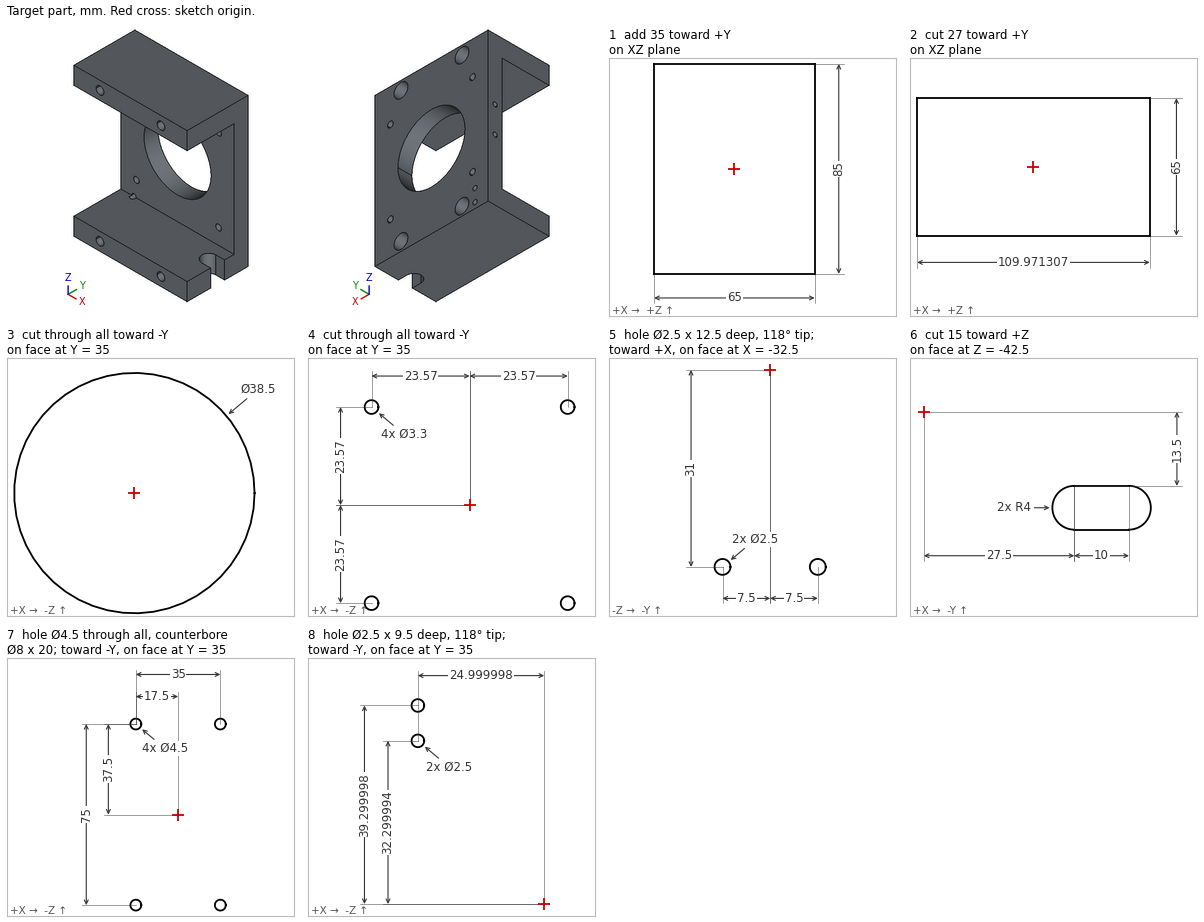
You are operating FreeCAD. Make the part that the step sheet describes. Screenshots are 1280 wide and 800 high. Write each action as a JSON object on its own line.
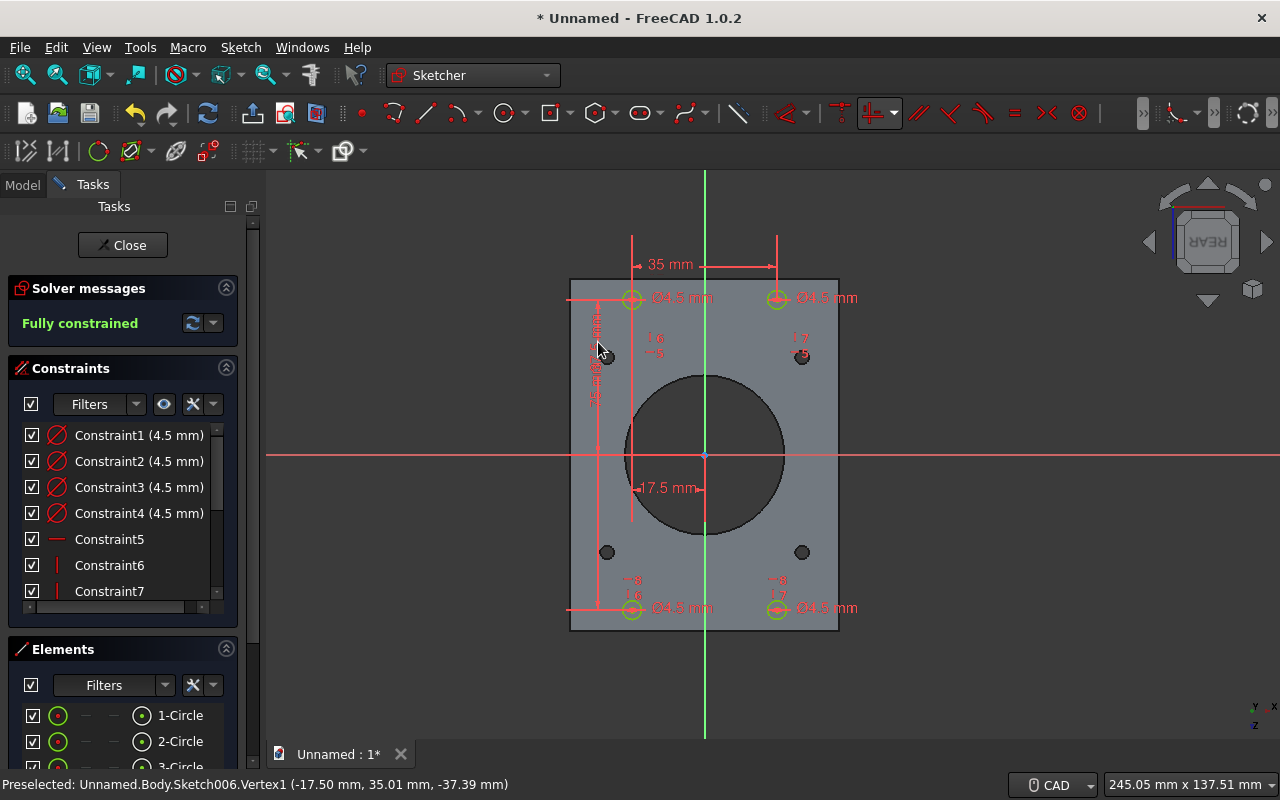
{"action": "left_click", "coordinate": [123, 245]}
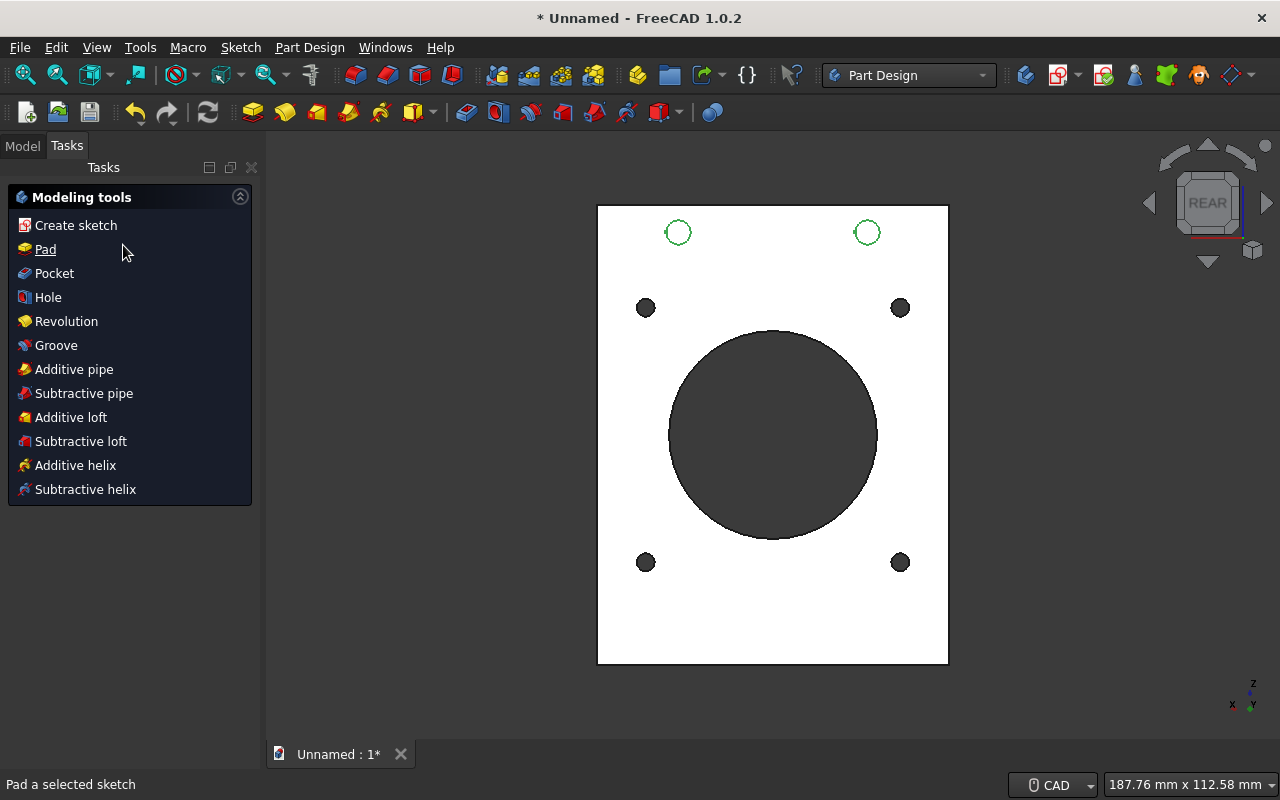
{"action": "left_click", "coordinate": [500, 112]}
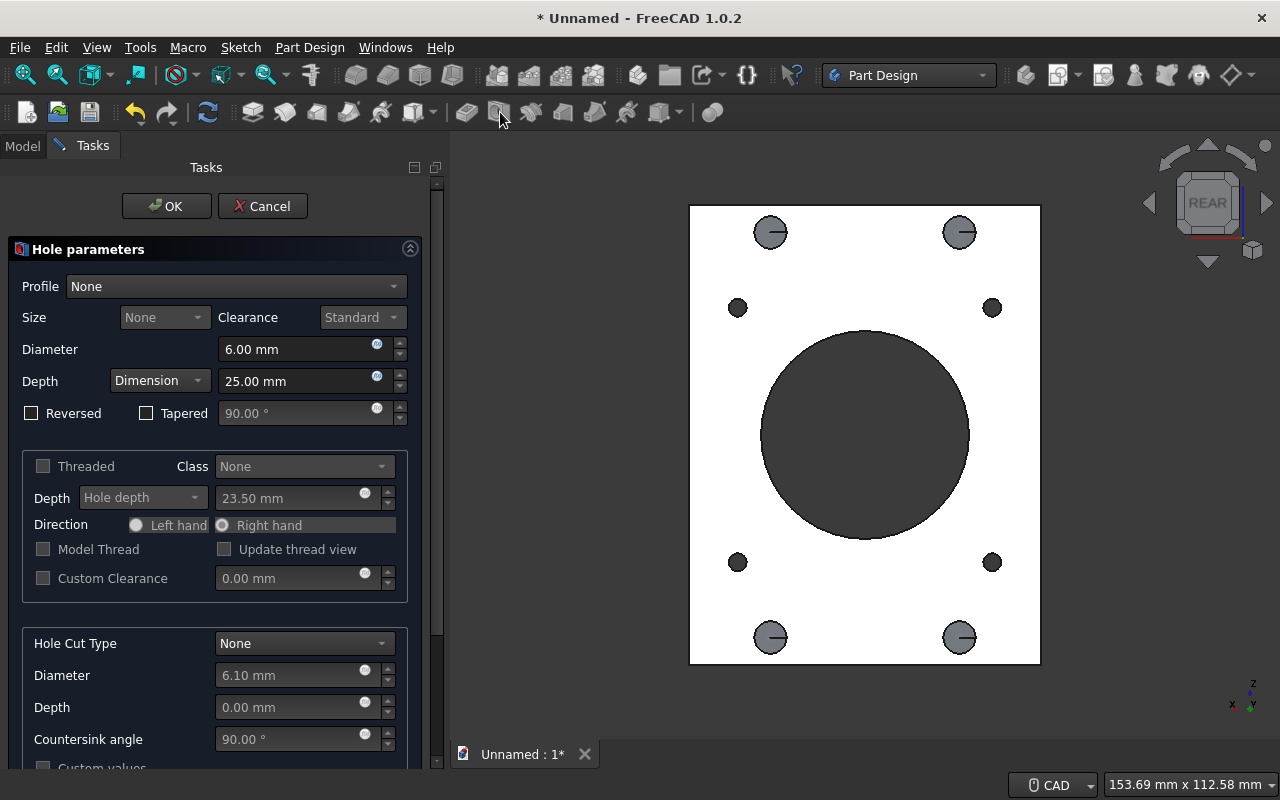
{"action": "triple_click", "coordinate": [305, 349]}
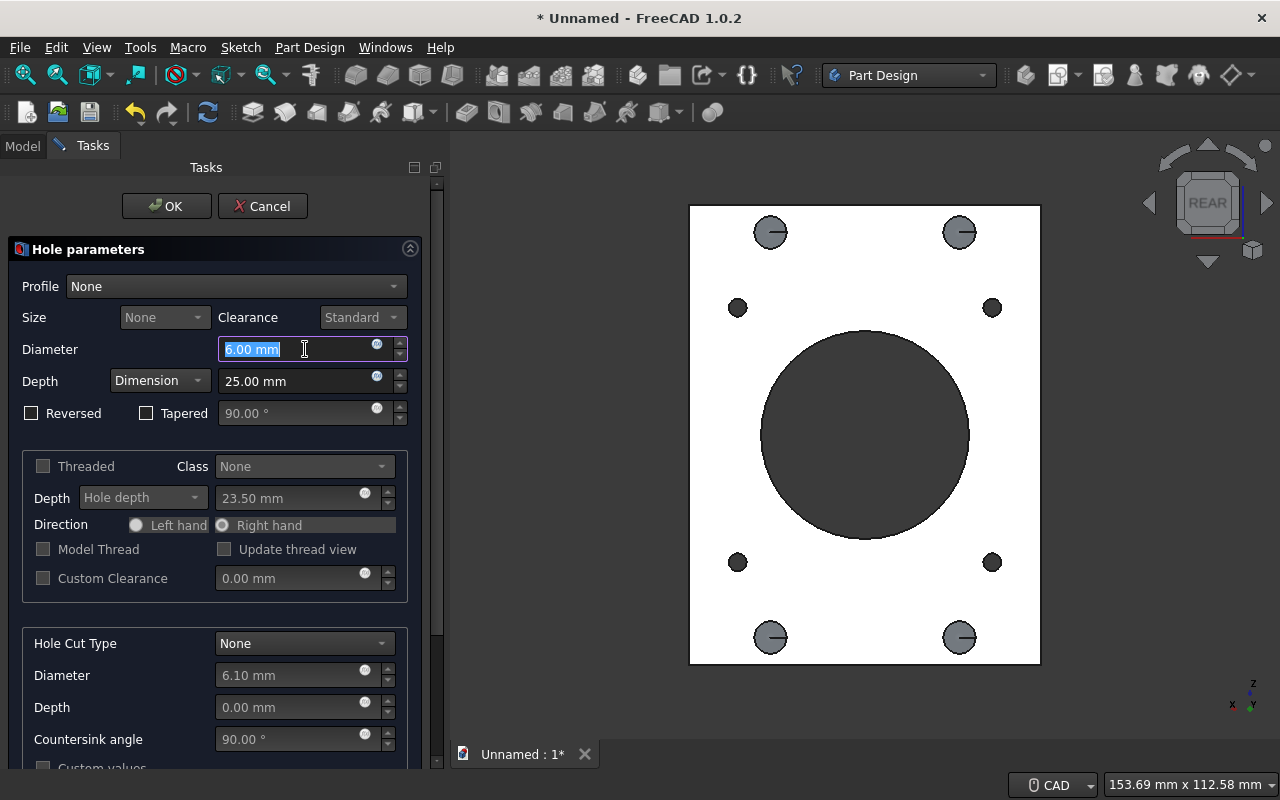
{"action": "type", "text": "4.5"}
{"action": "key", "text": "Tab"}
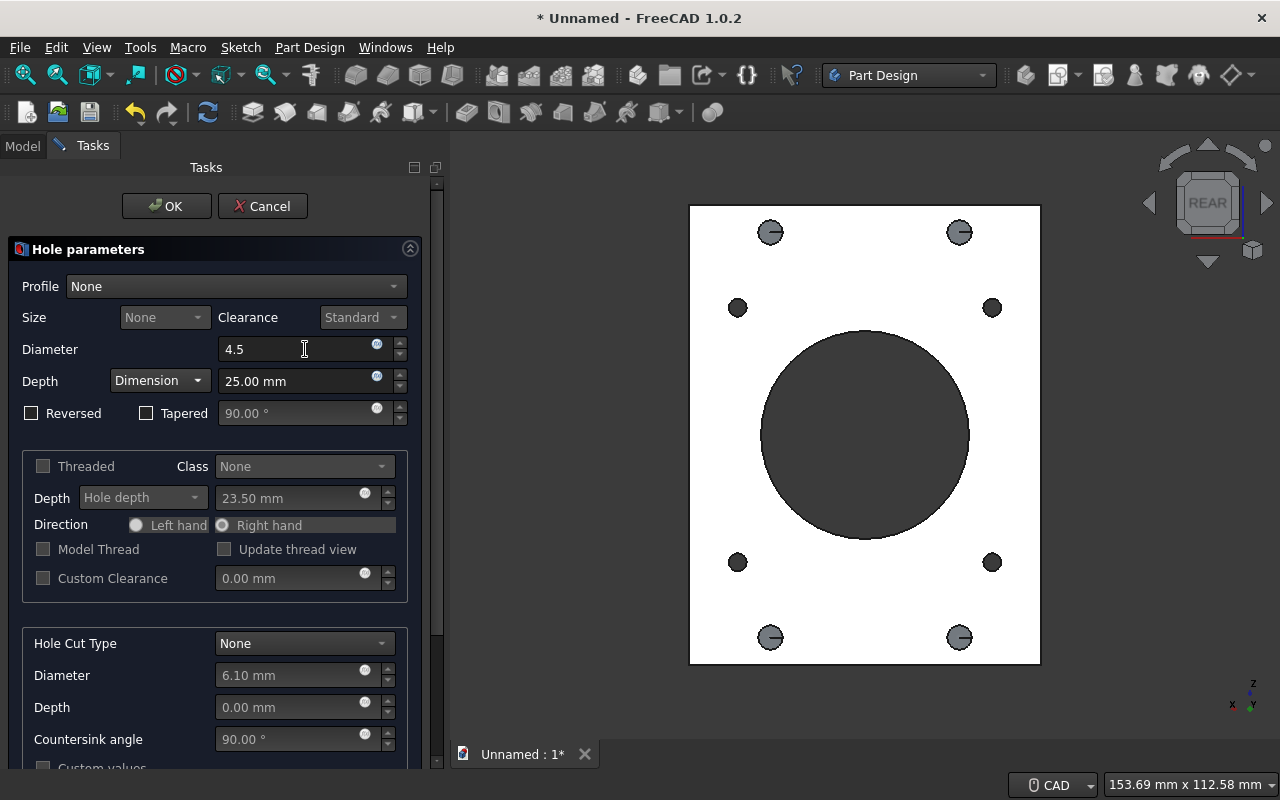
{"action": "left_click", "coordinate": [161, 380]}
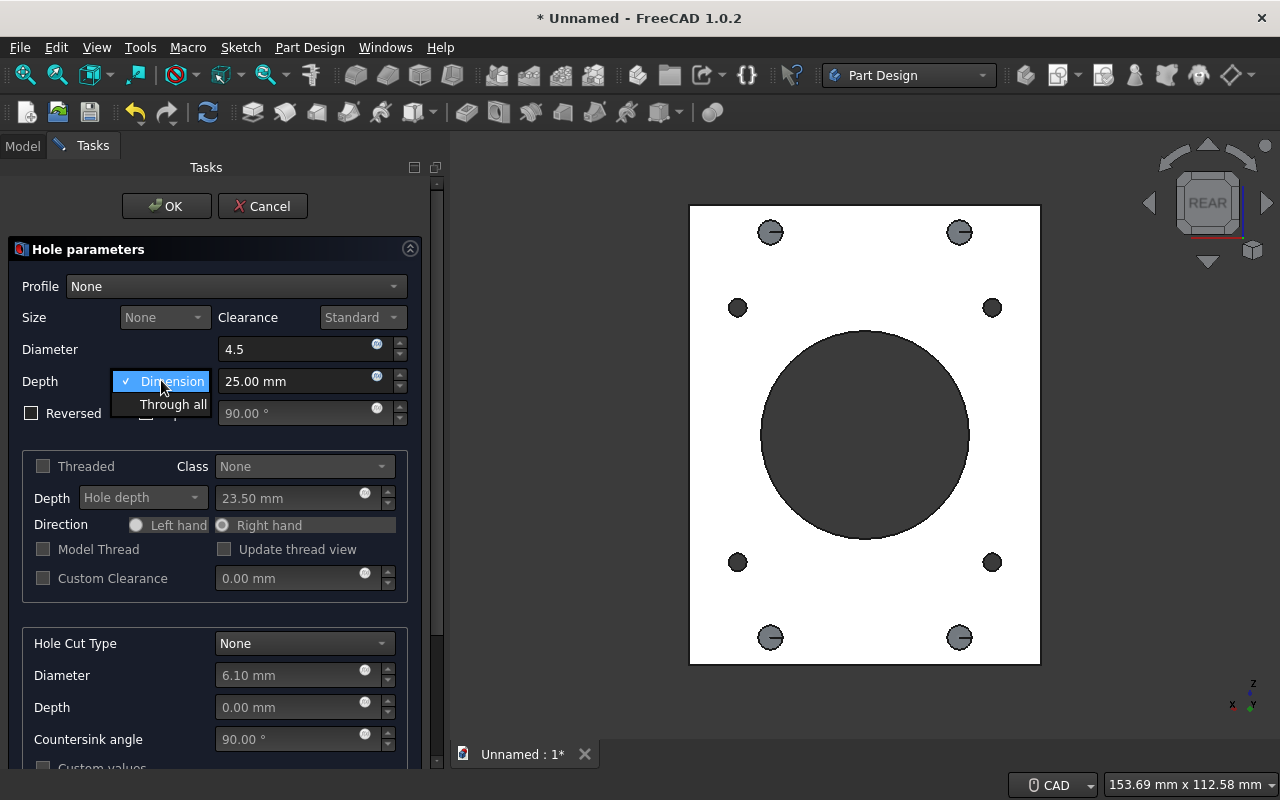
{"action": "left_click", "coordinate": [160, 404]}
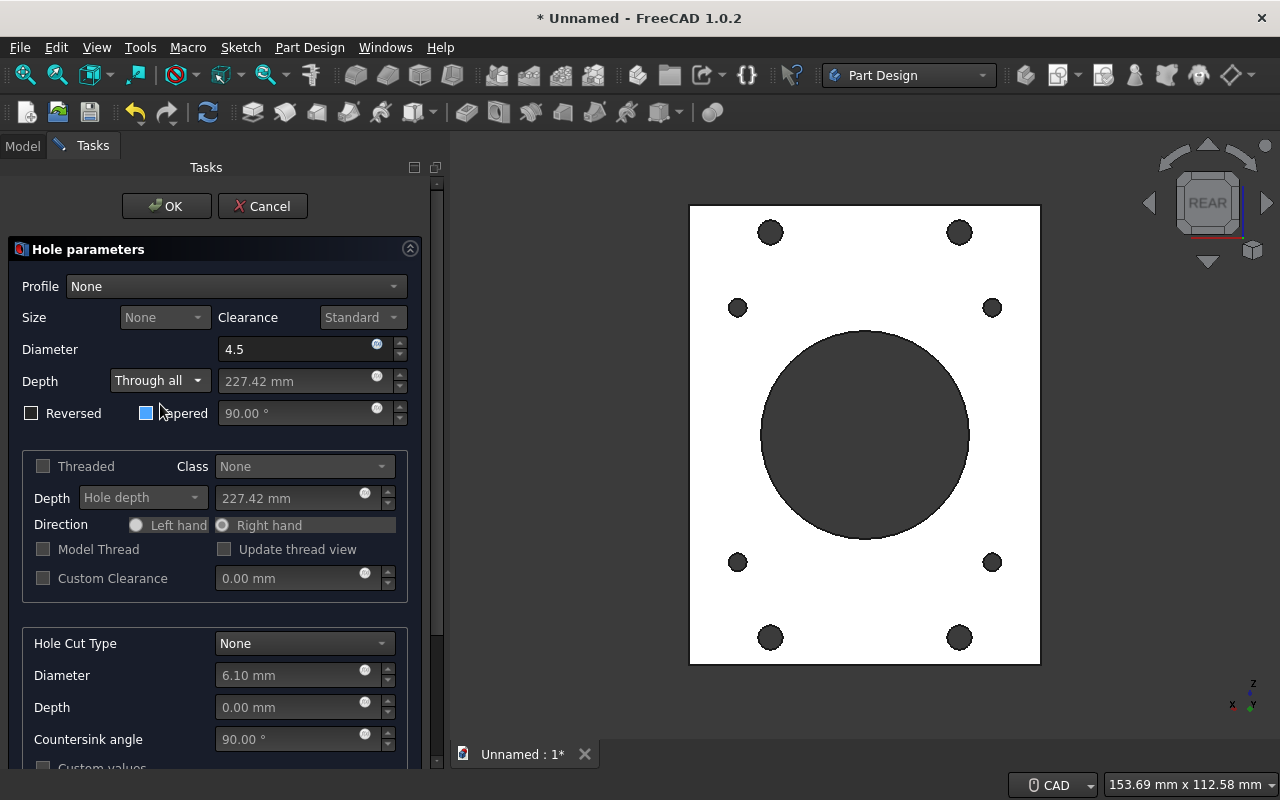
{"action": "left_click", "coordinate": [306, 644]}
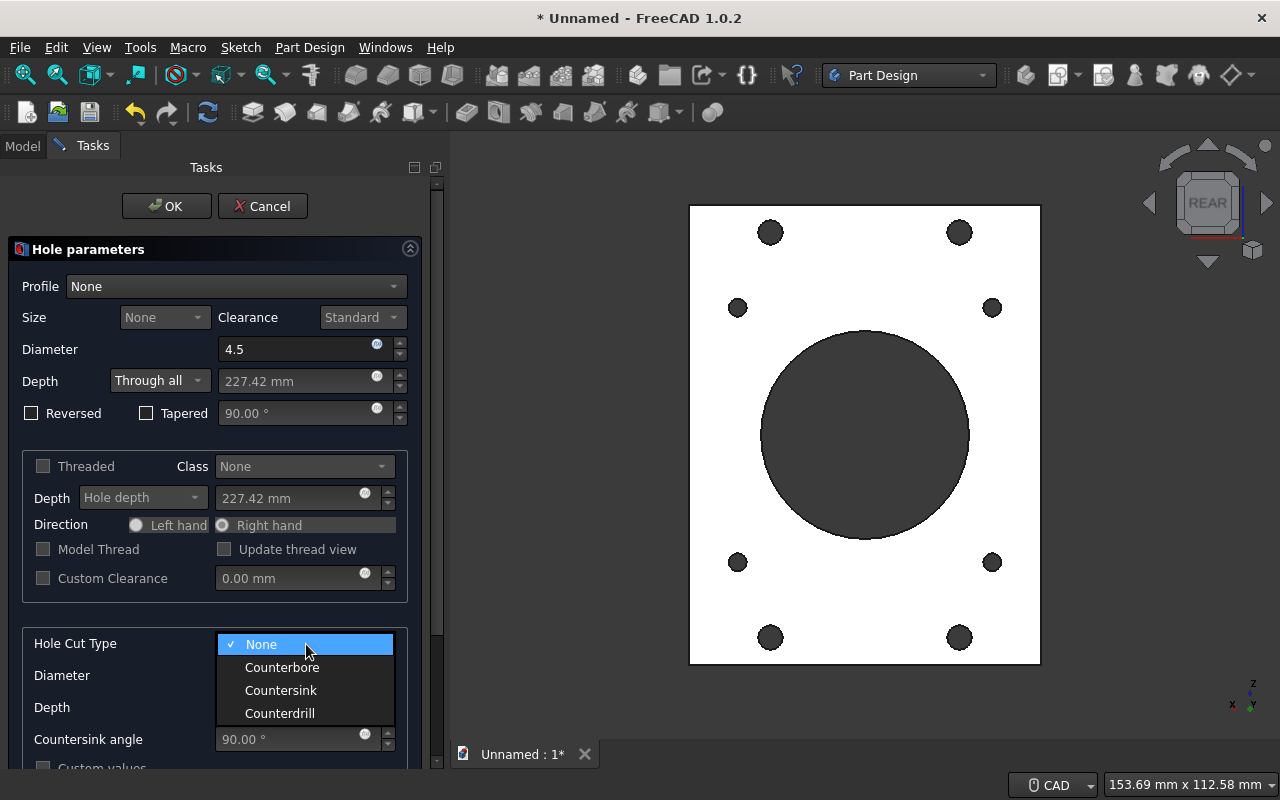
{"action": "left_click", "coordinate": [304, 668]}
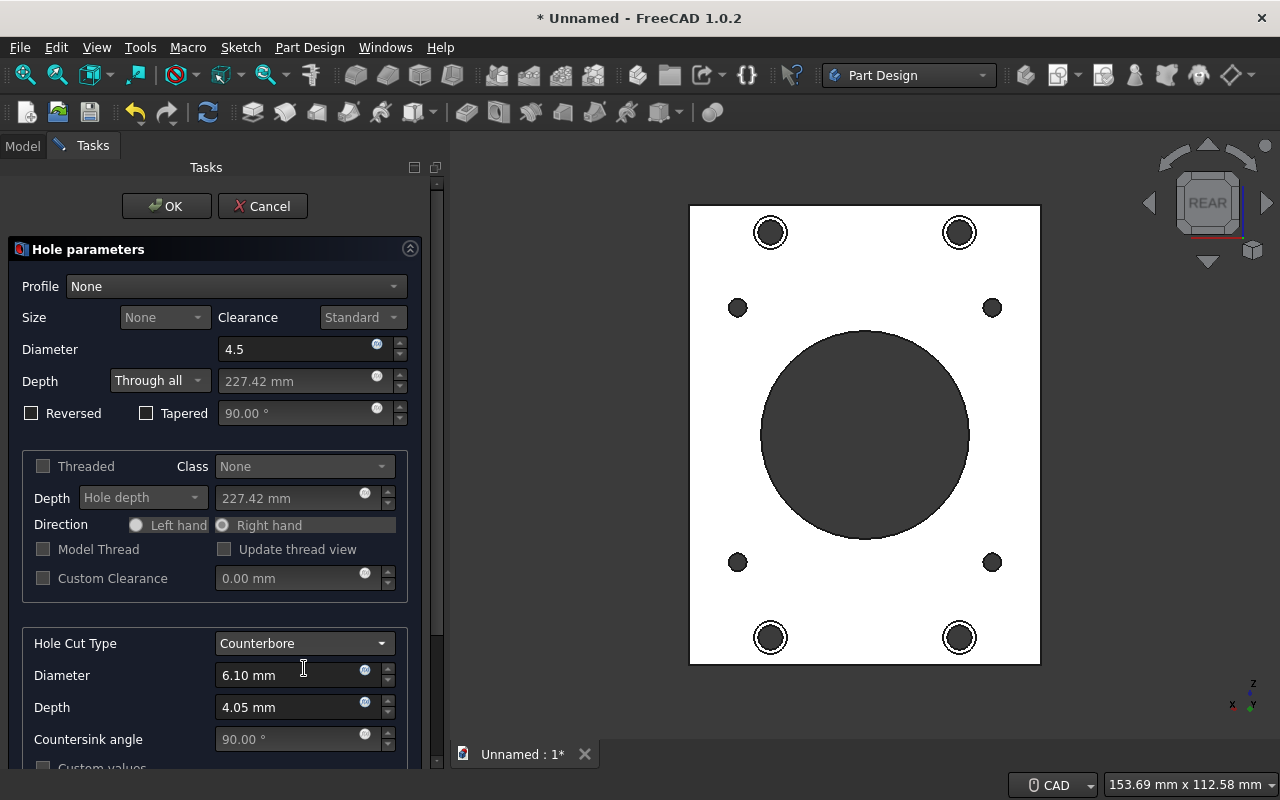
{"action": "triple_click", "coordinate": [298, 675]}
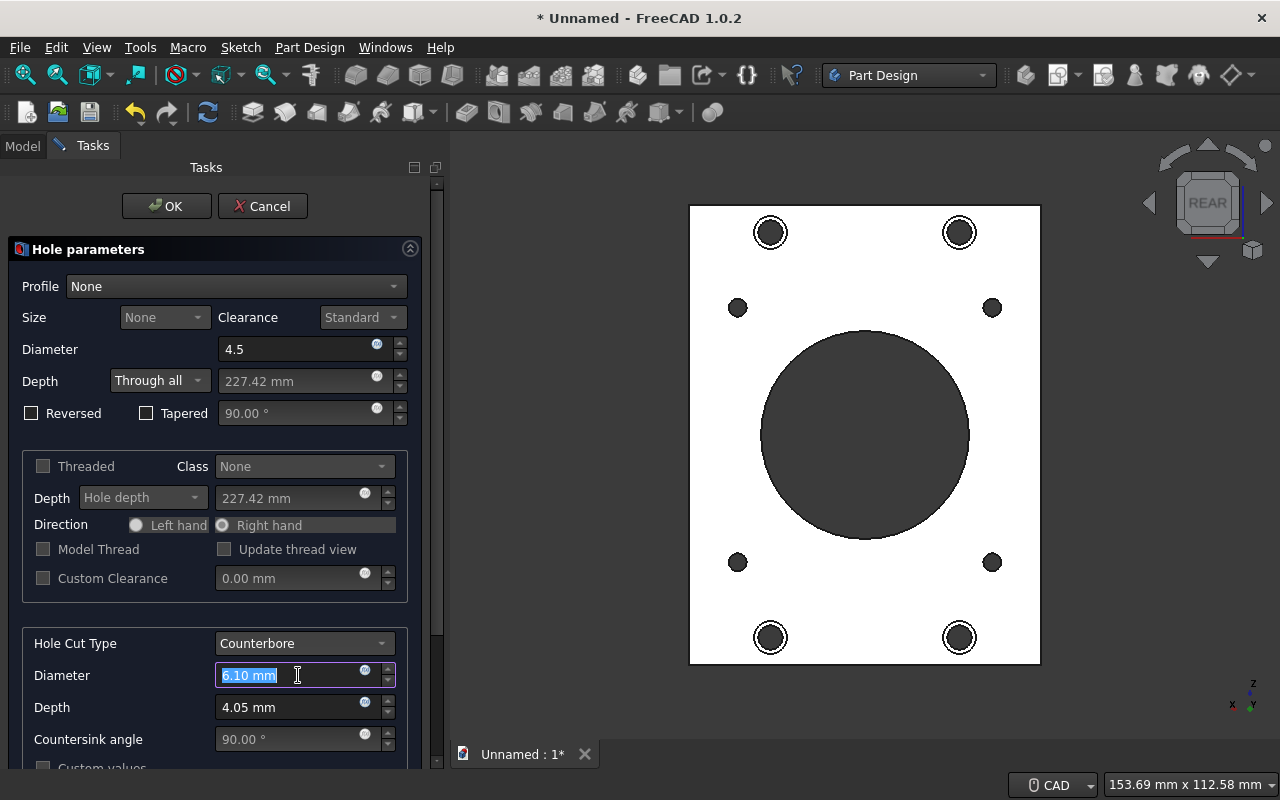
{"action": "type", "text": "8"}
{"action": "key", "text": "Tab"}